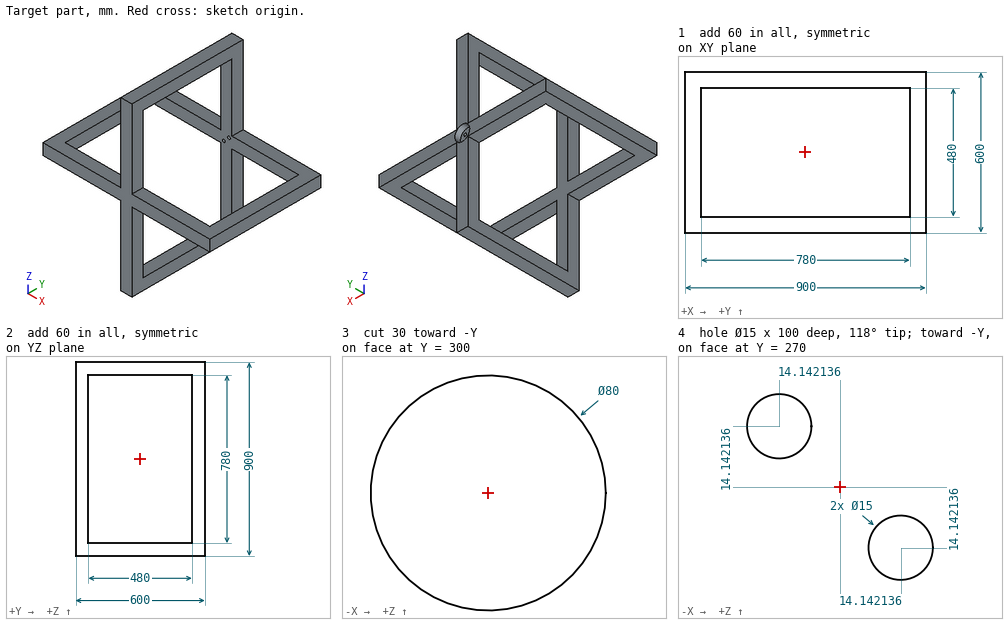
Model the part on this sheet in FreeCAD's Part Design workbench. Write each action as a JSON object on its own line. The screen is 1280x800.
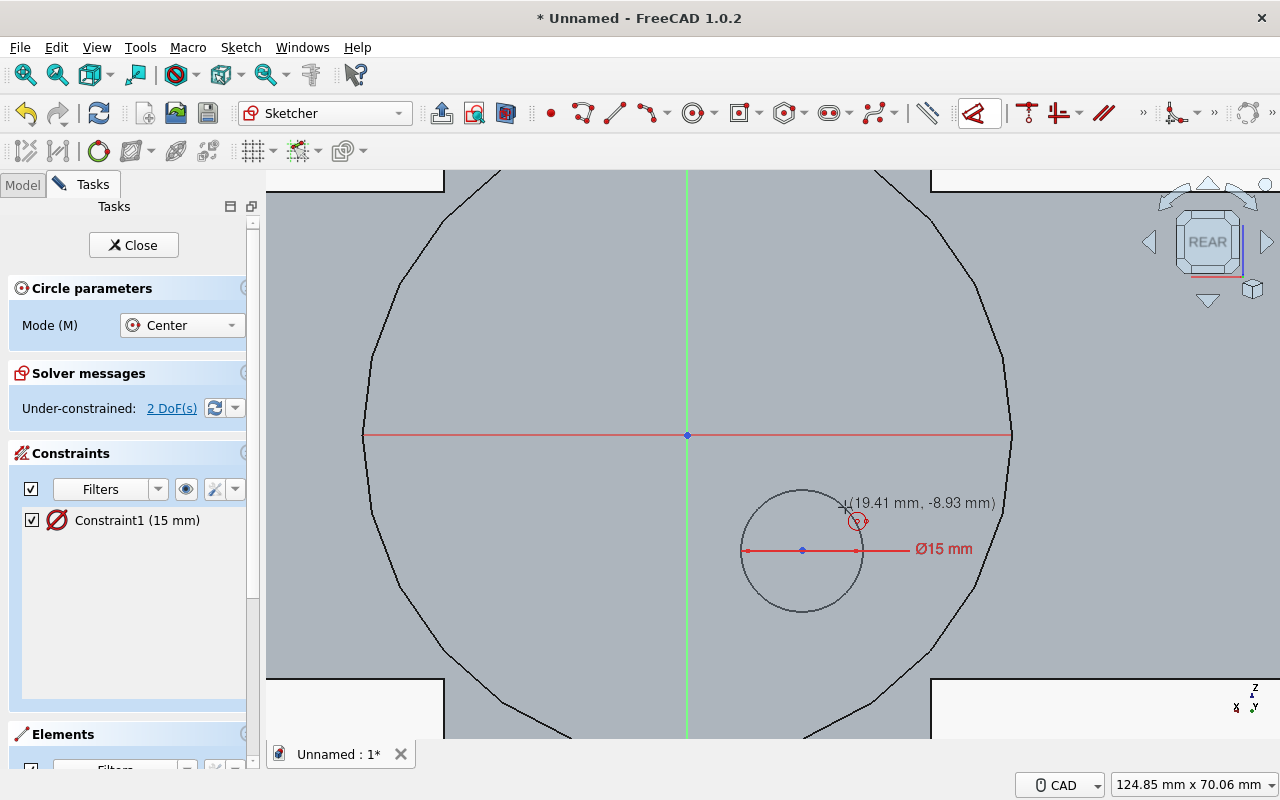
{"action": "left_click", "coordinate": [572, 321]}
{"action": "mouse_move", "coordinate": [616, 278]}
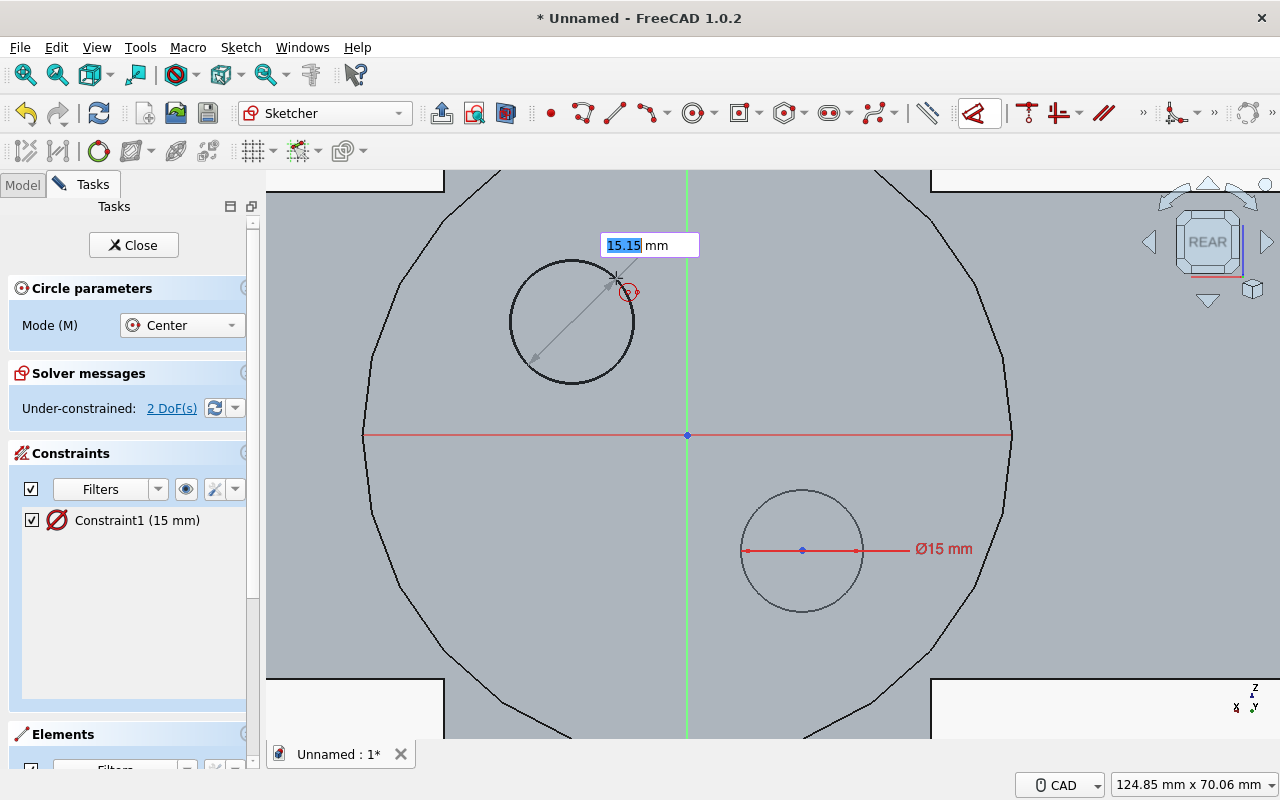
{"action": "type", "text": "15"}
{"action": "key", "text": "Return"}
{"action": "key", "text": "Escape"}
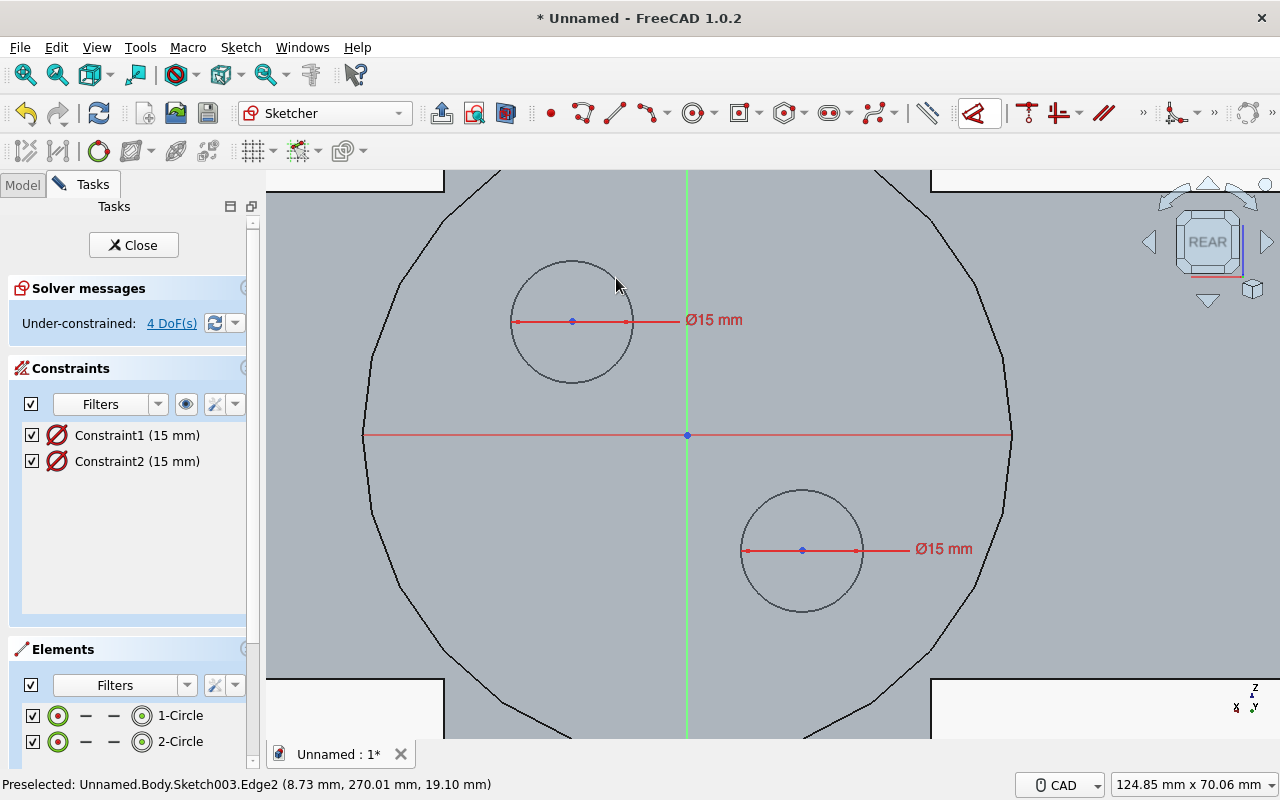
{"action": "left_click", "coordinate": [974, 114]}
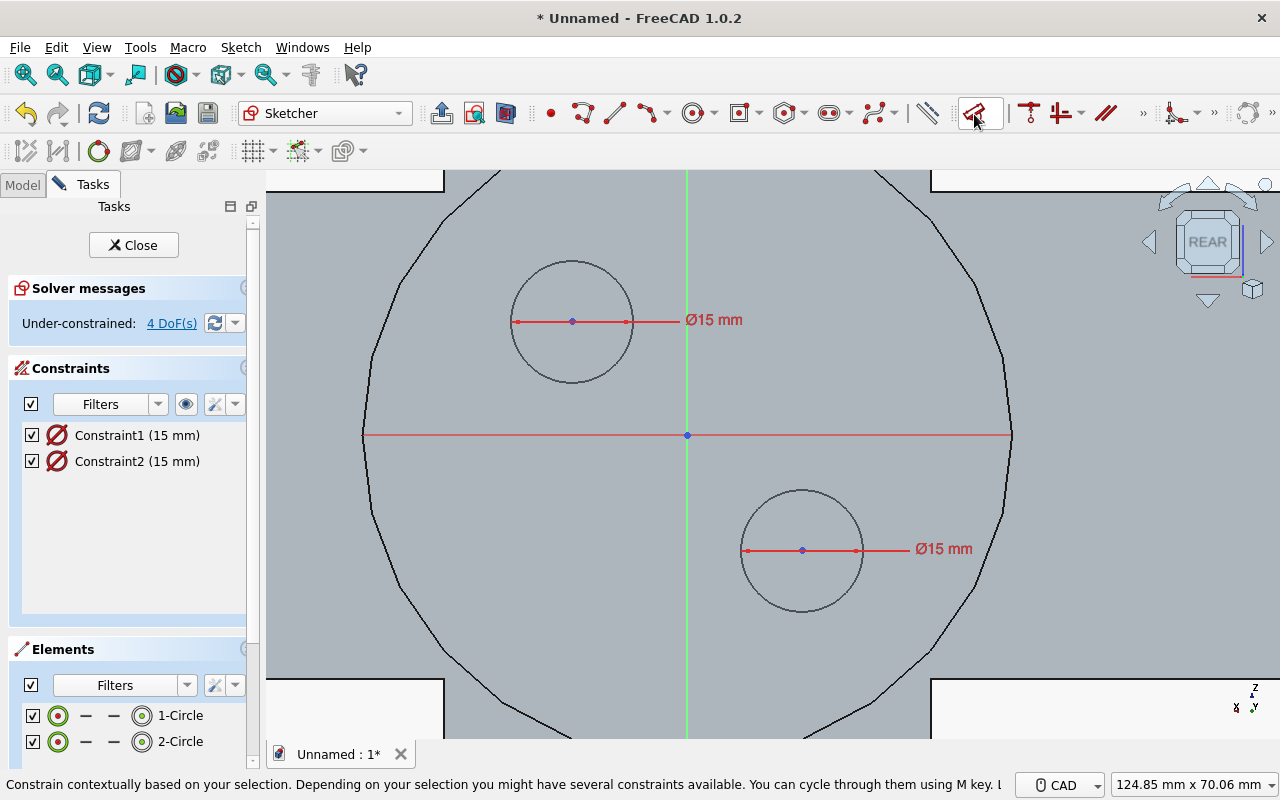
{"action": "left_click", "coordinate": [802, 551]}
{"action": "left_click", "coordinate": [718, 585]}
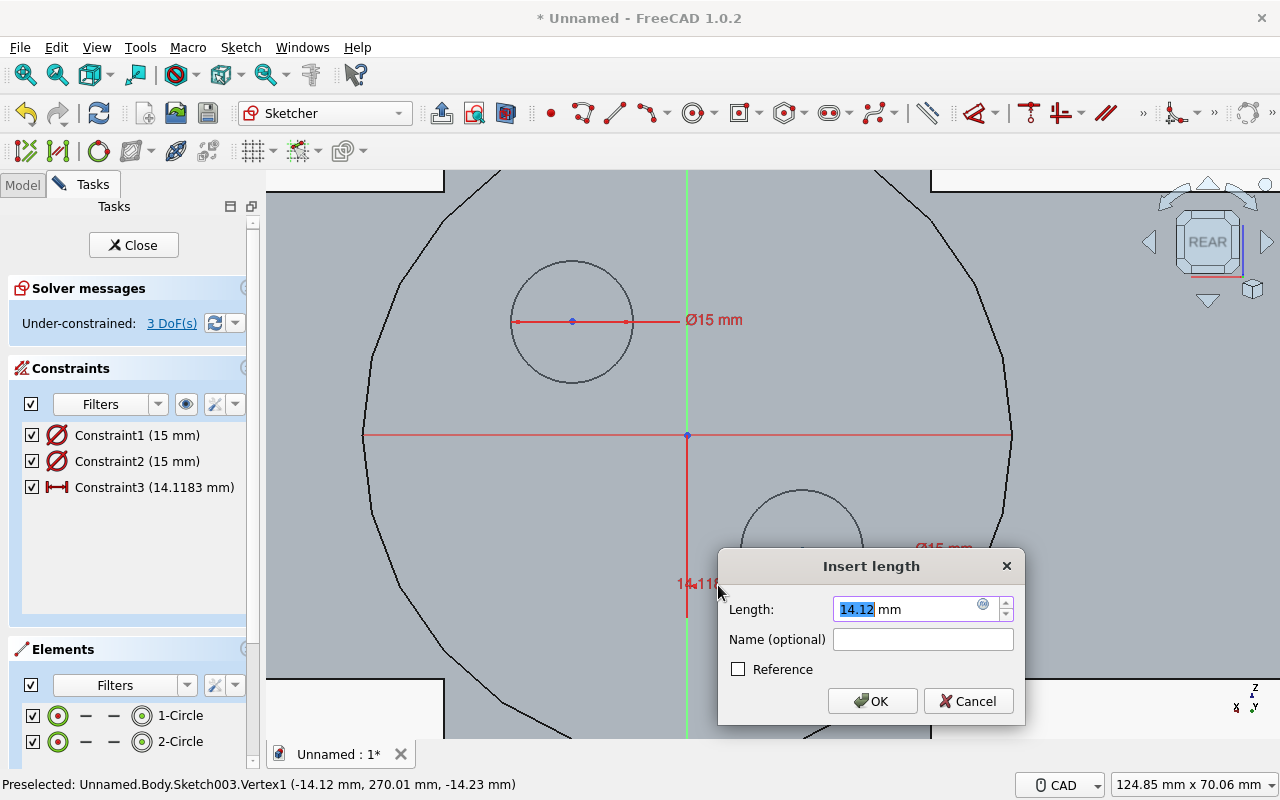
{"action": "type", "text": "14.142136"}
{"action": "key", "text": "Return"}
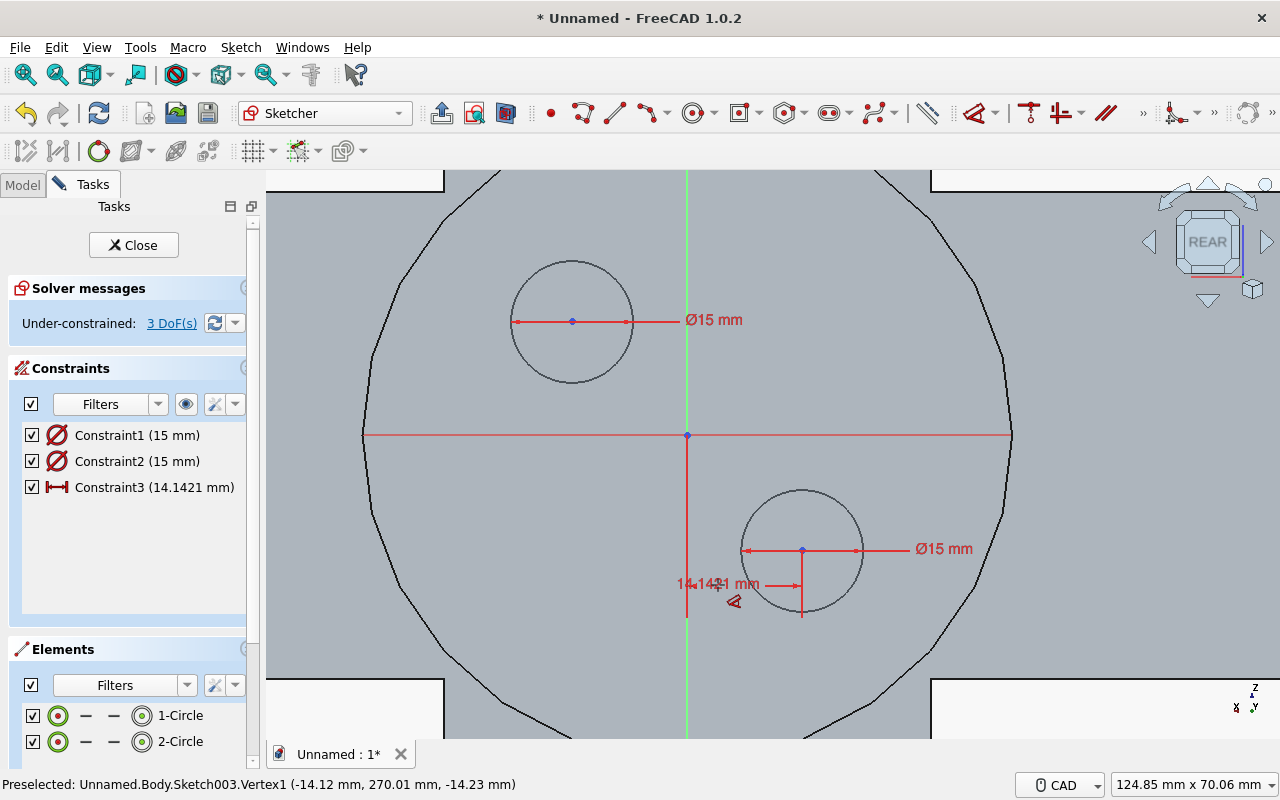
{"action": "left_click", "coordinate": [802, 551]}
{"action": "left_click", "coordinate": [836, 467]}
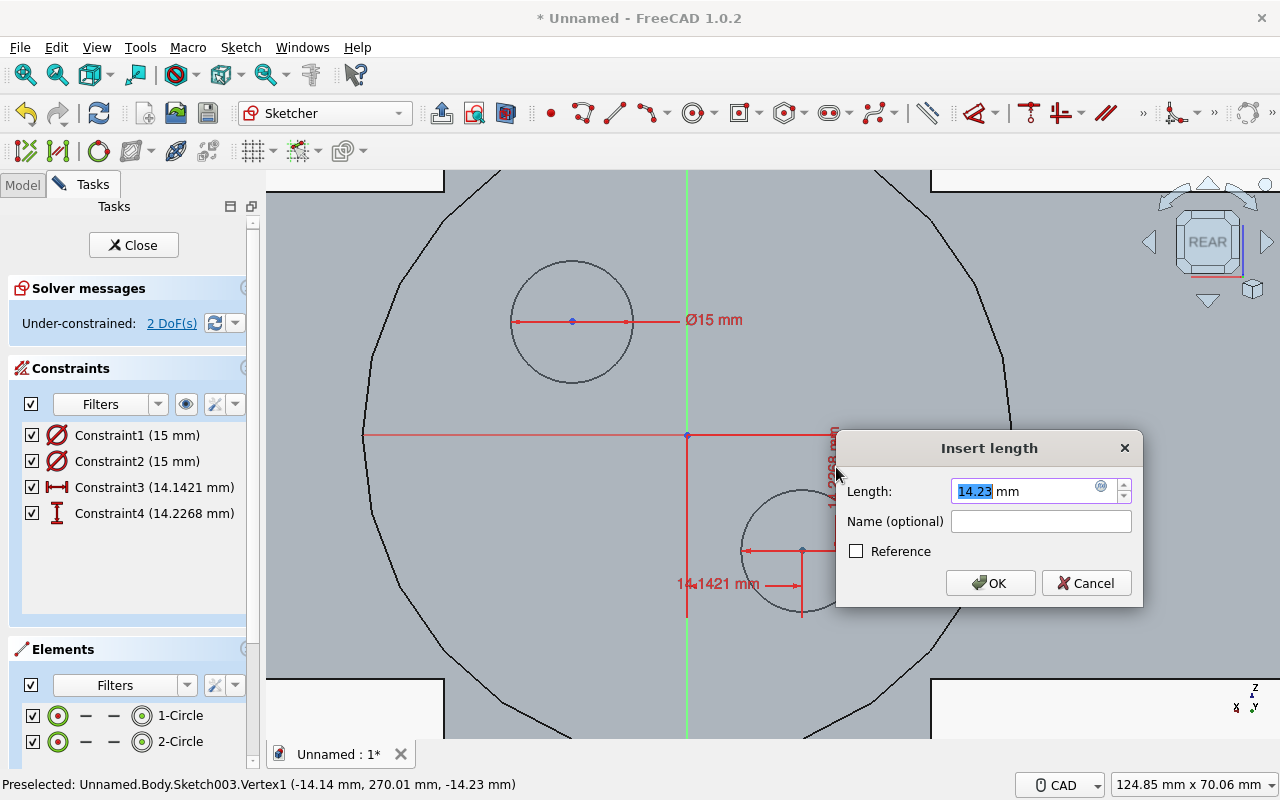
{"action": "type", "text": "14.142136"}
{"action": "key", "text": "Return"}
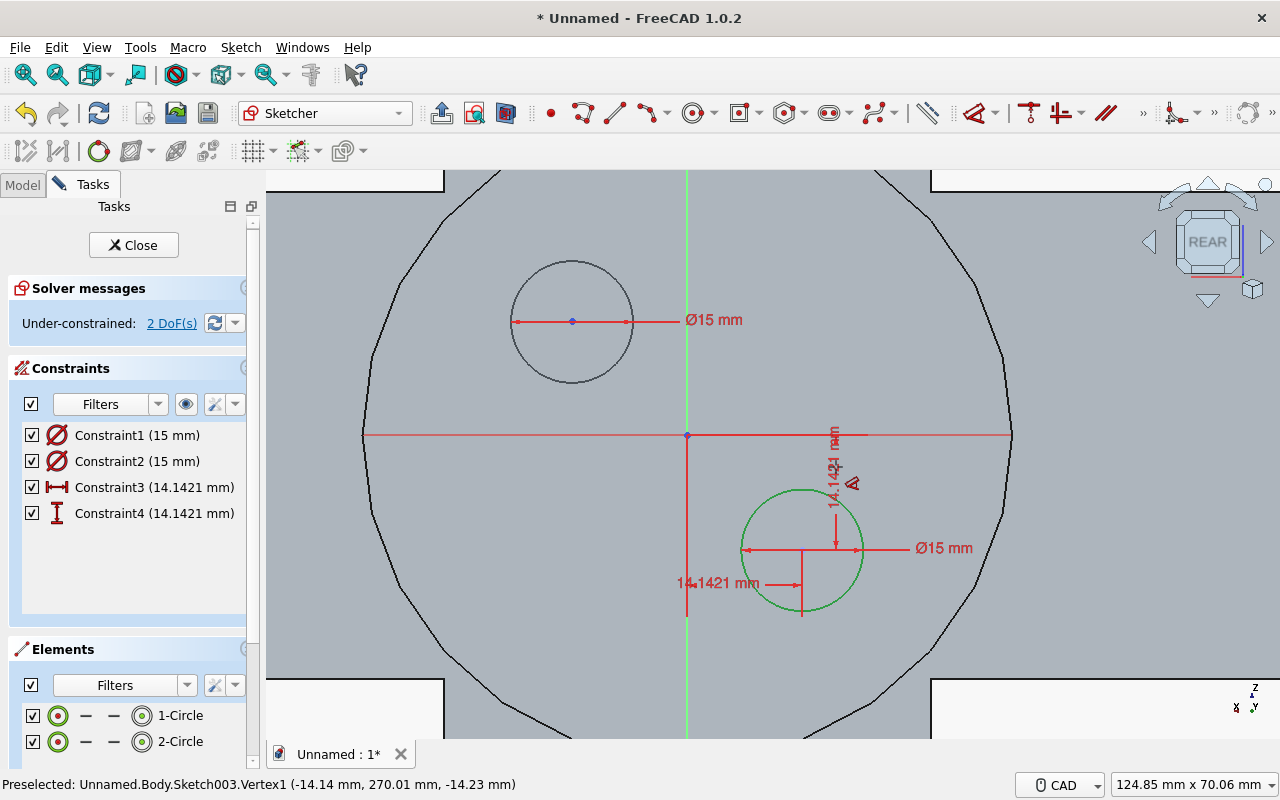
{"action": "left_click", "coordinate": [572, 322]}
{"action": "left_click", "coordinate": [603, 288]}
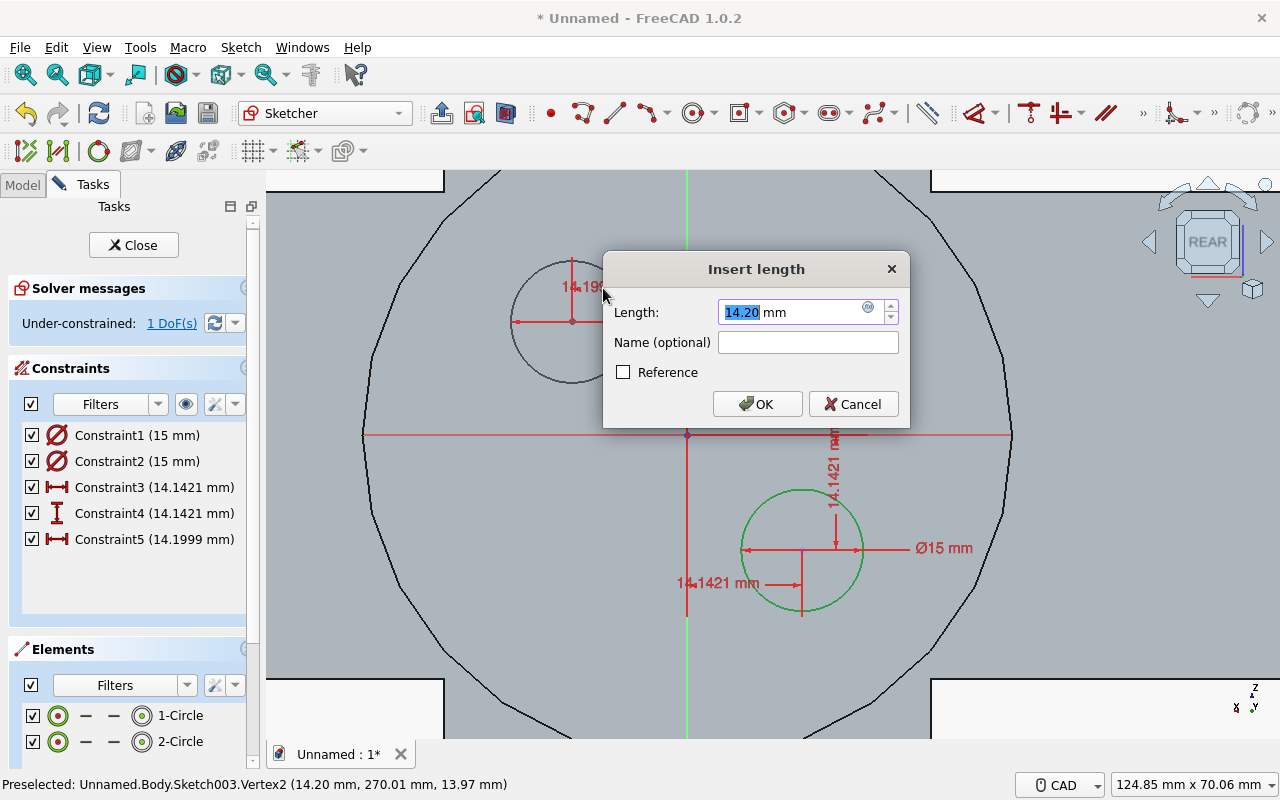
{"action": "type", "text": "14.142136"}
{"action": "key", "text": "Return"}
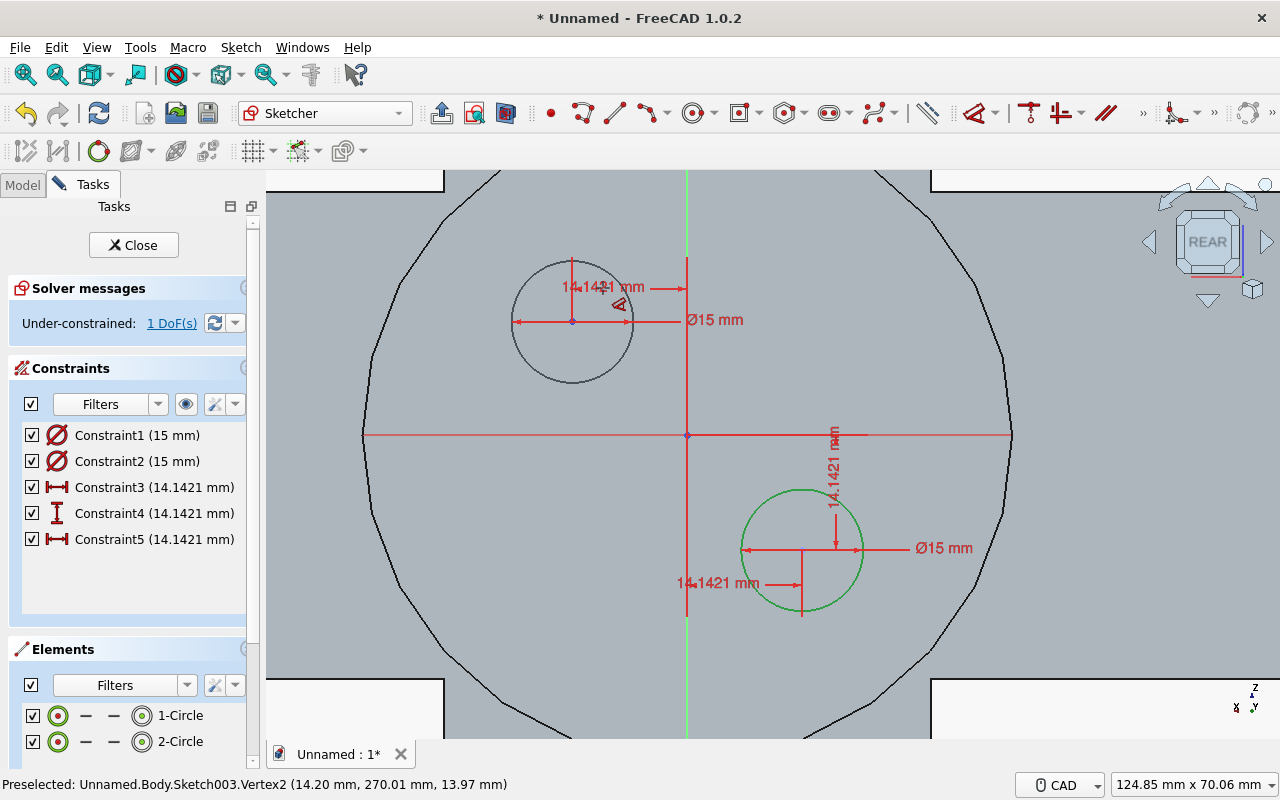
{"action": "left_click", "coordinate": [572, 322]}
{"action": "left_click", "coordinate": [538, 353]}